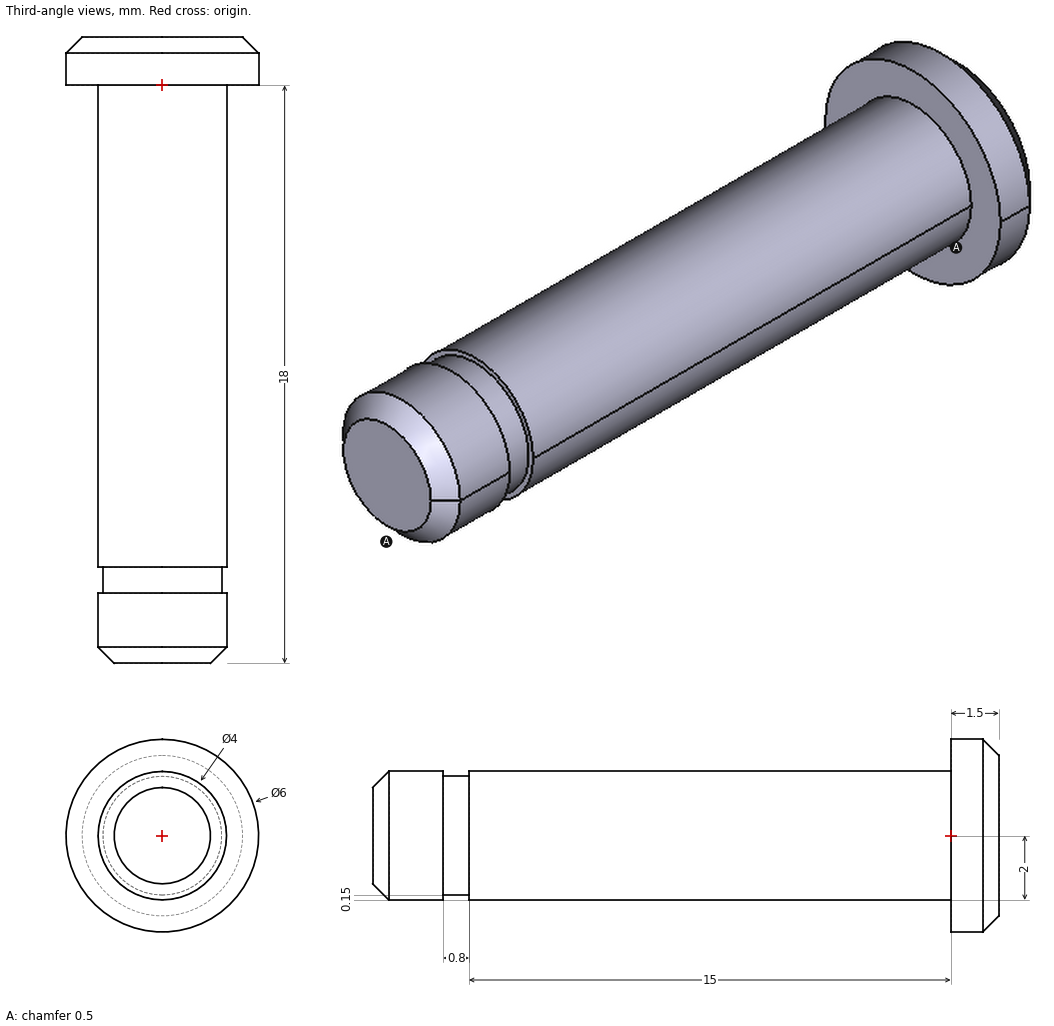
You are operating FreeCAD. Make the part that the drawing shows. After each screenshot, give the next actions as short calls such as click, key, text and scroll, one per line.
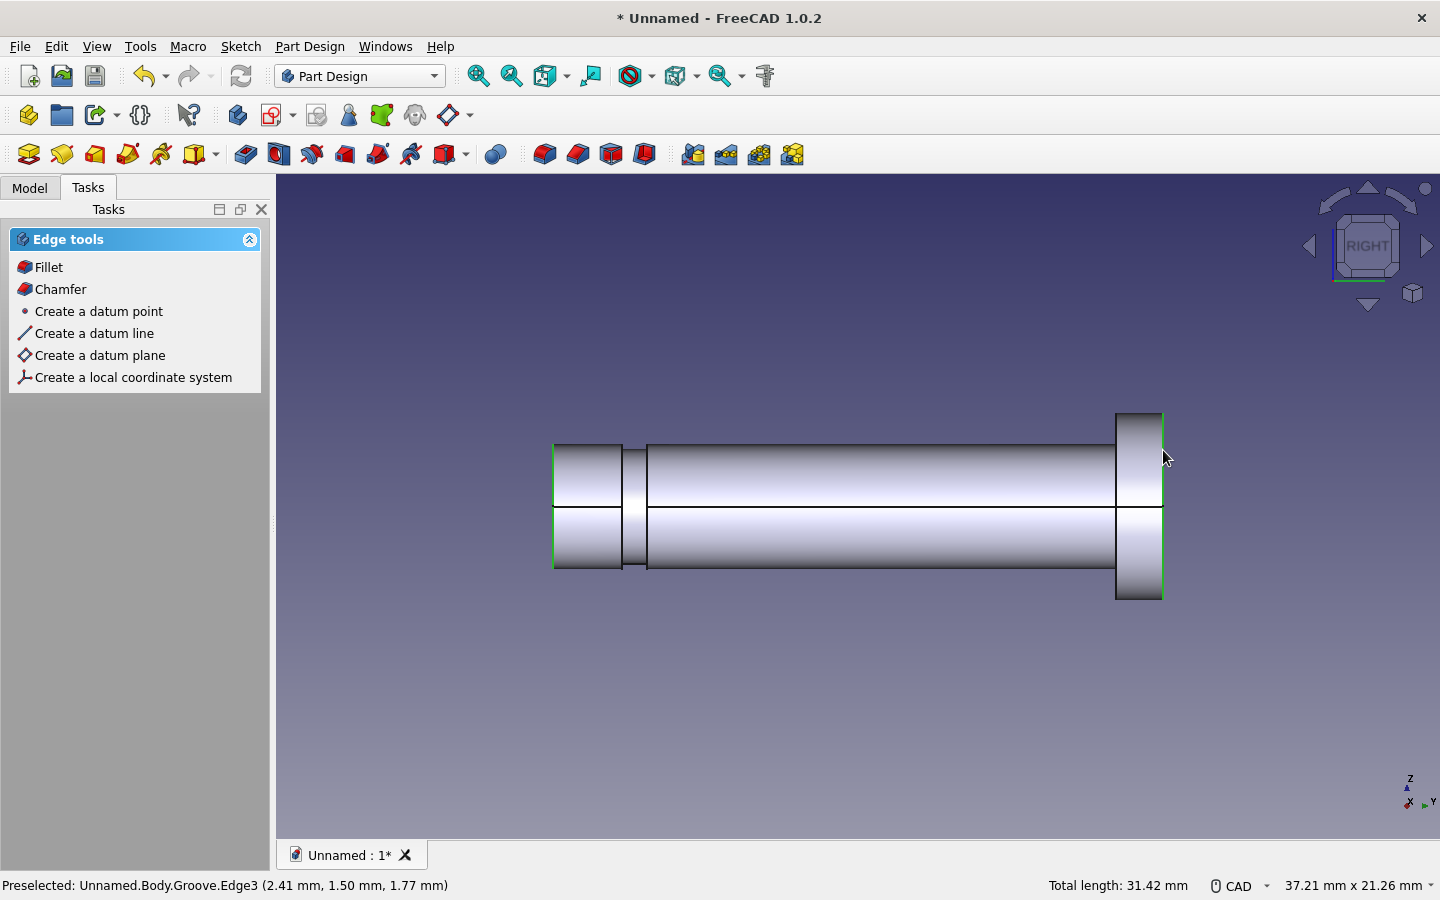
click(578, 154)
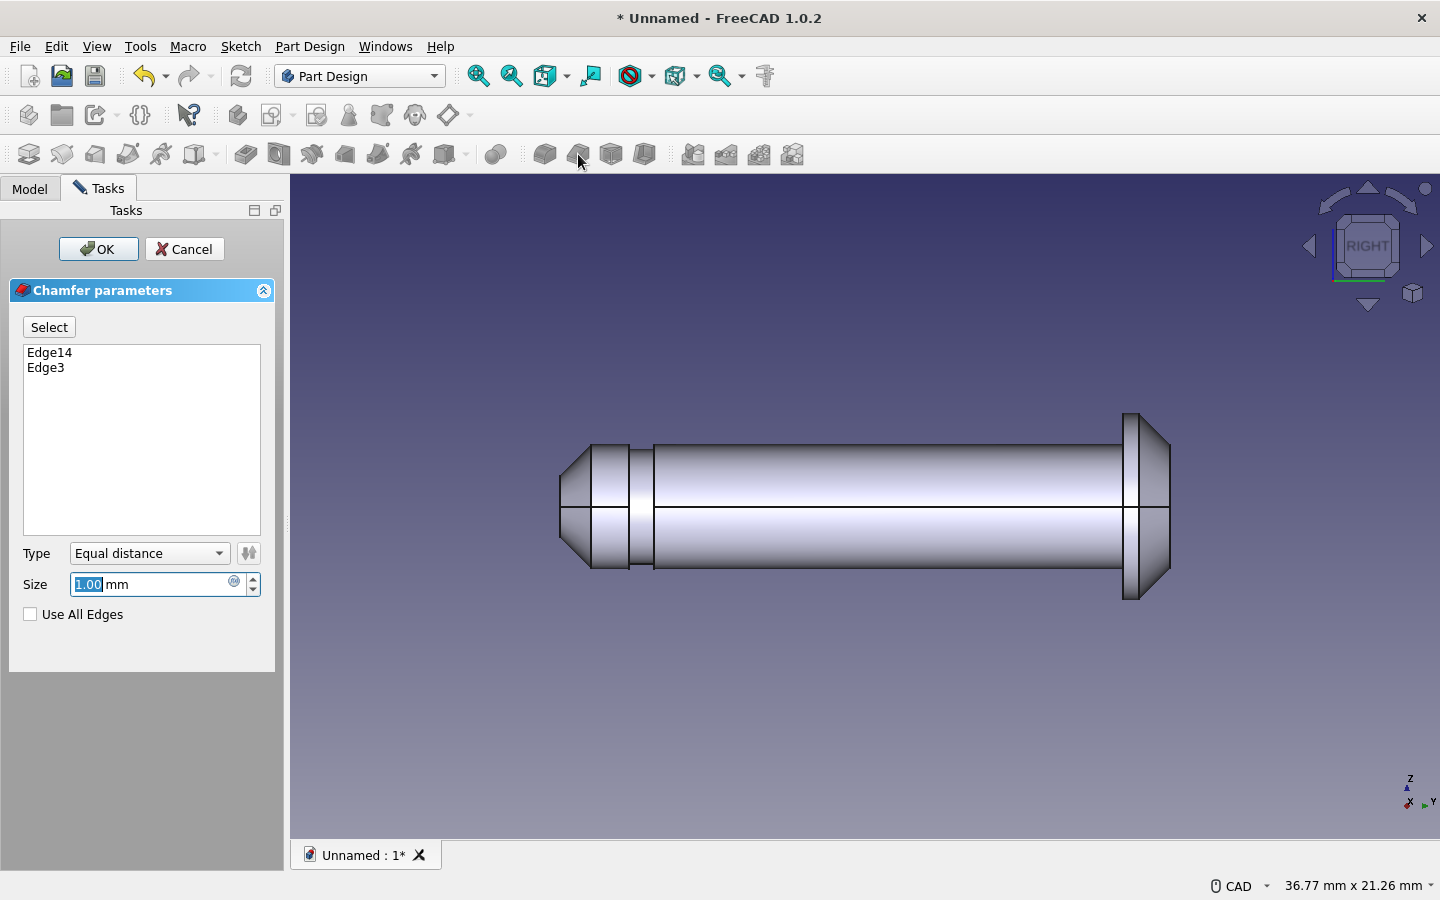
text(0.5)
key(Tab)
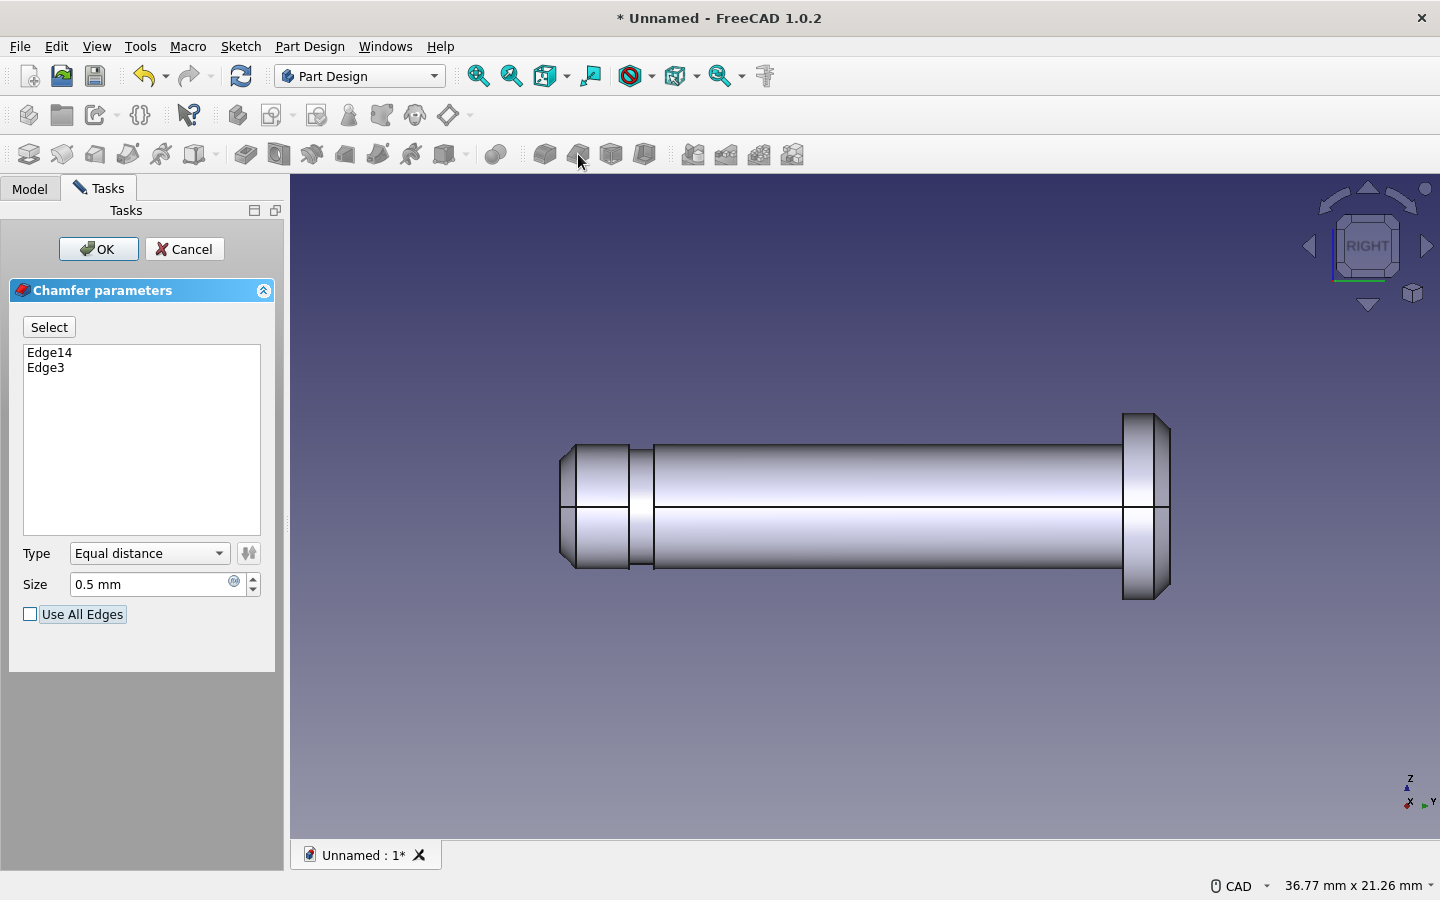
click(99, 249)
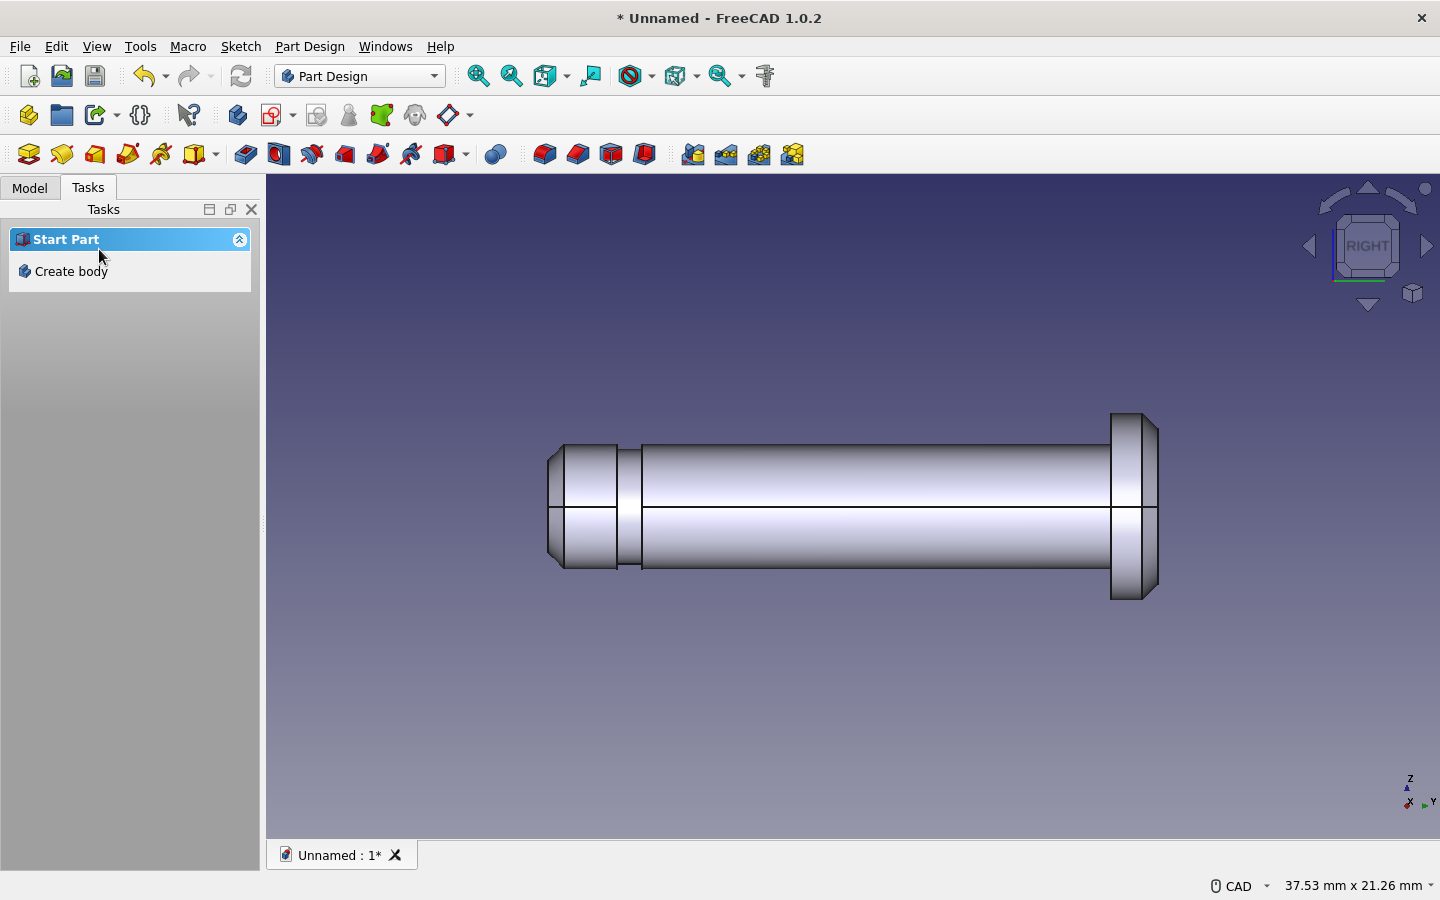
key(0)